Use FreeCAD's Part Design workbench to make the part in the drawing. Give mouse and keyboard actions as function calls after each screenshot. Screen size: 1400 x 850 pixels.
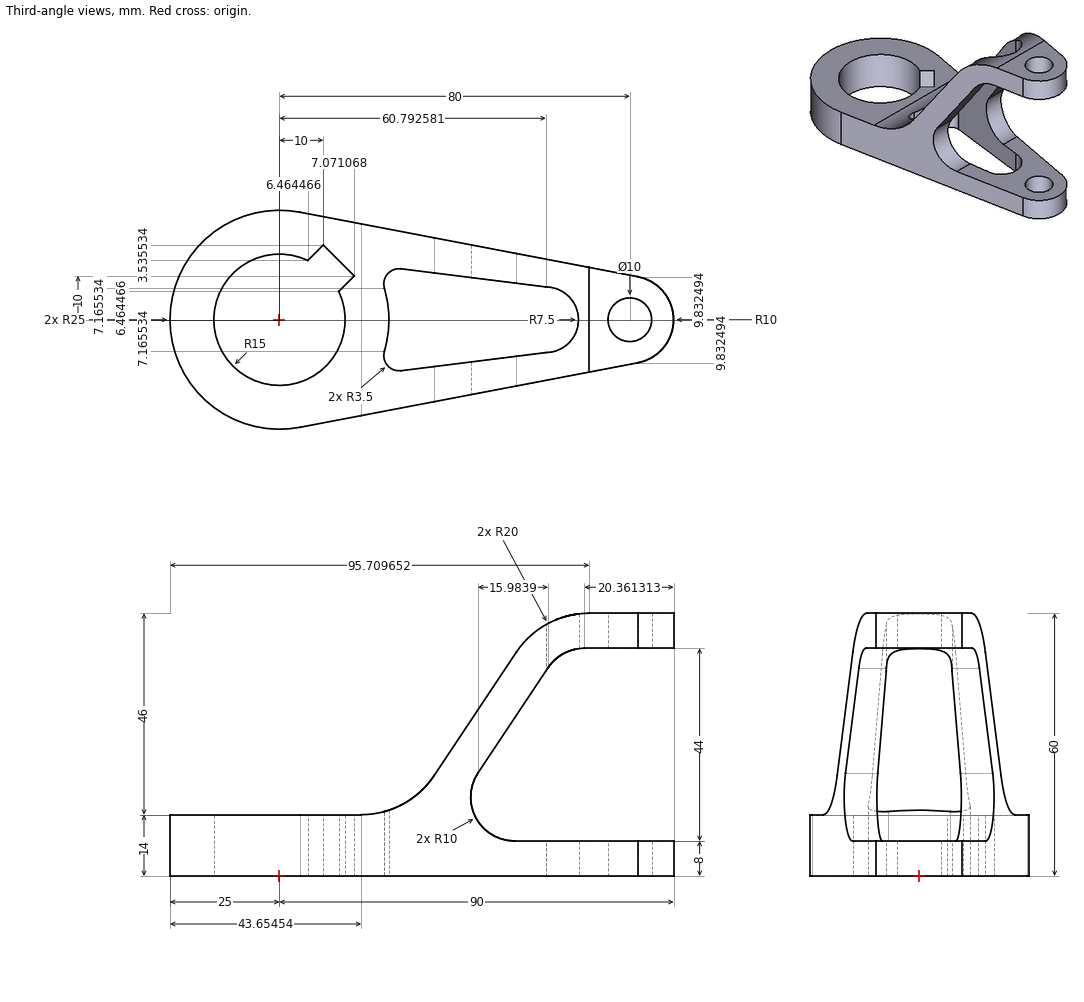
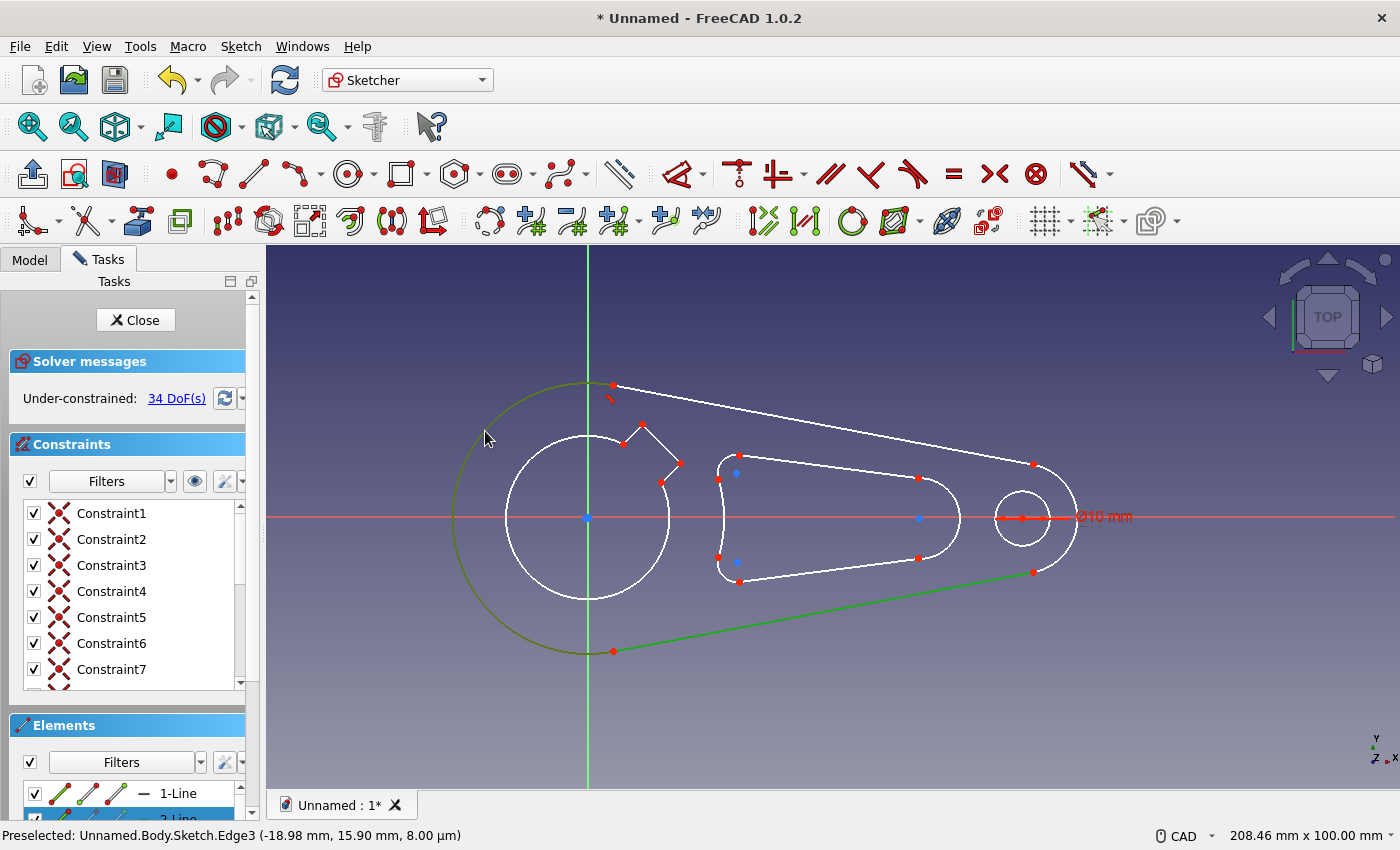
click(913, 174)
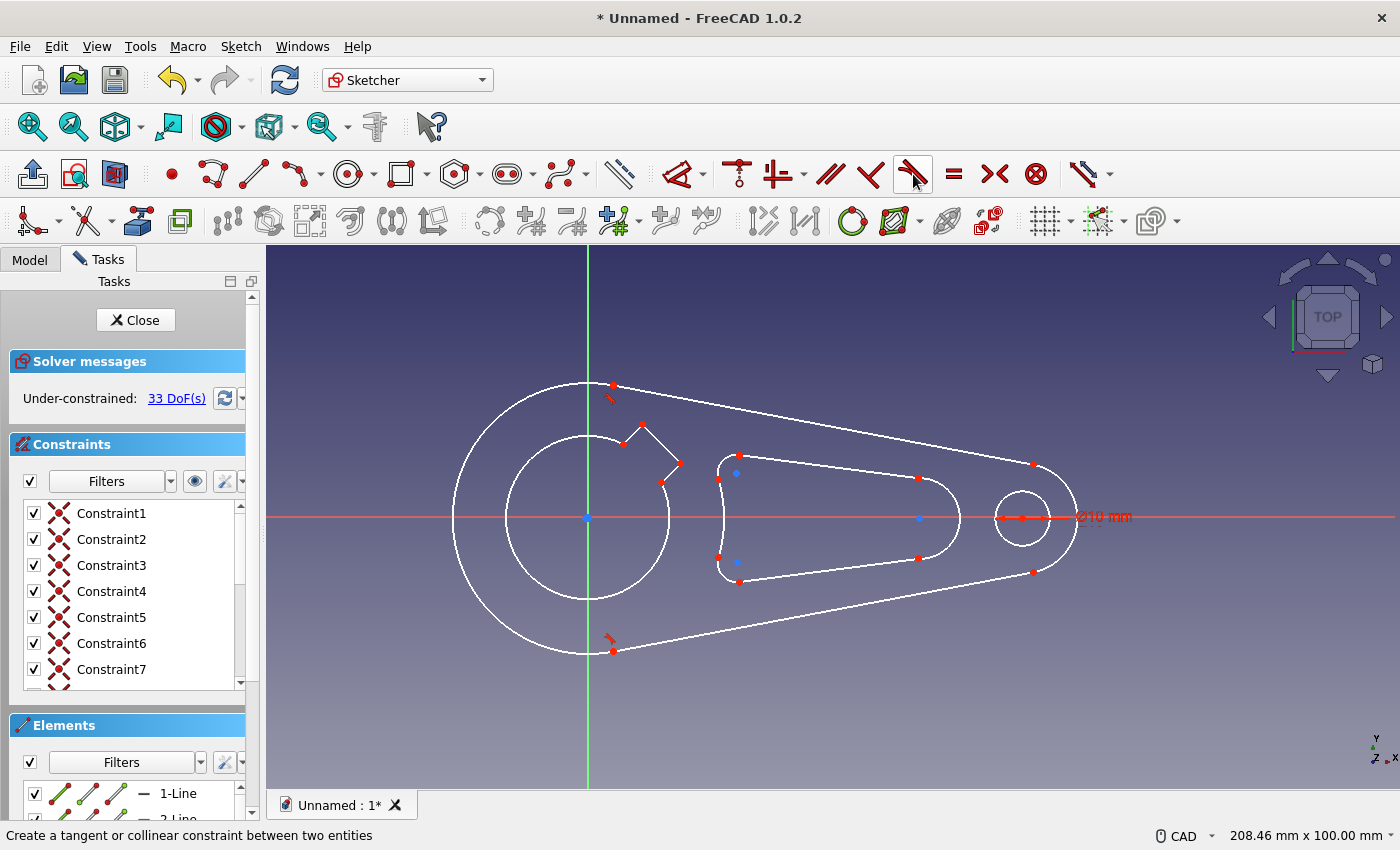
click(793, 462)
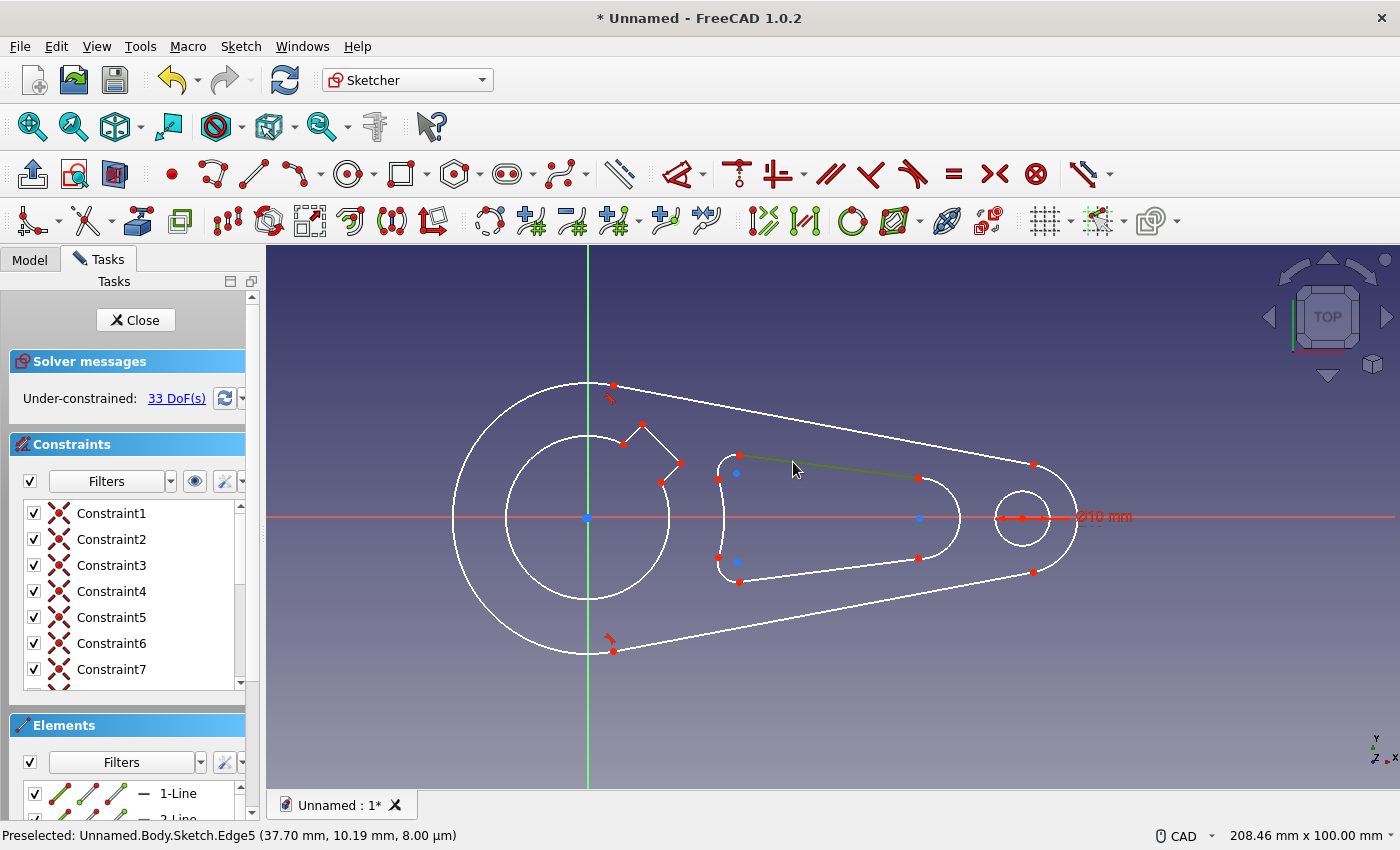
scroll(728, 457, up, 2)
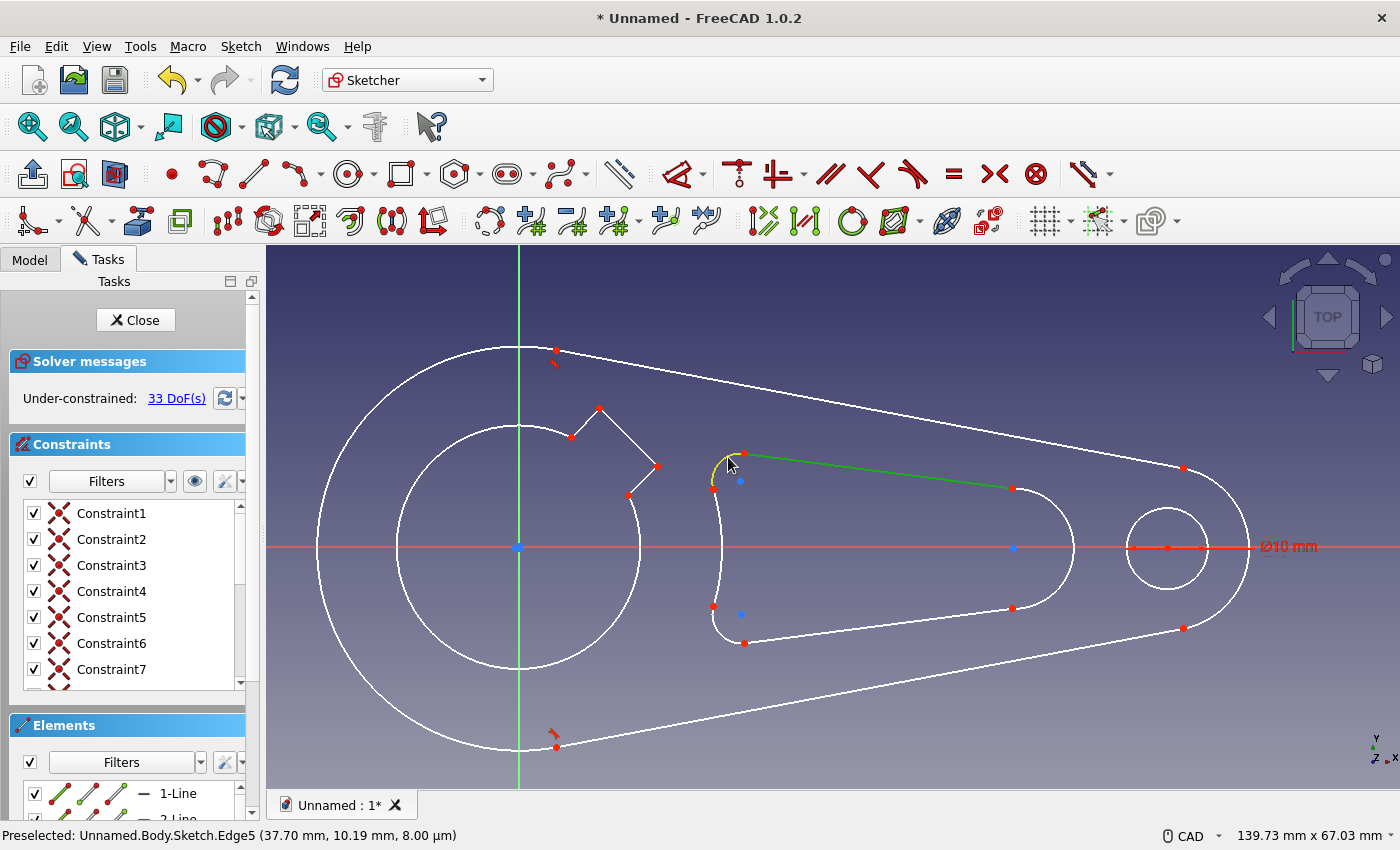
click(728, 456)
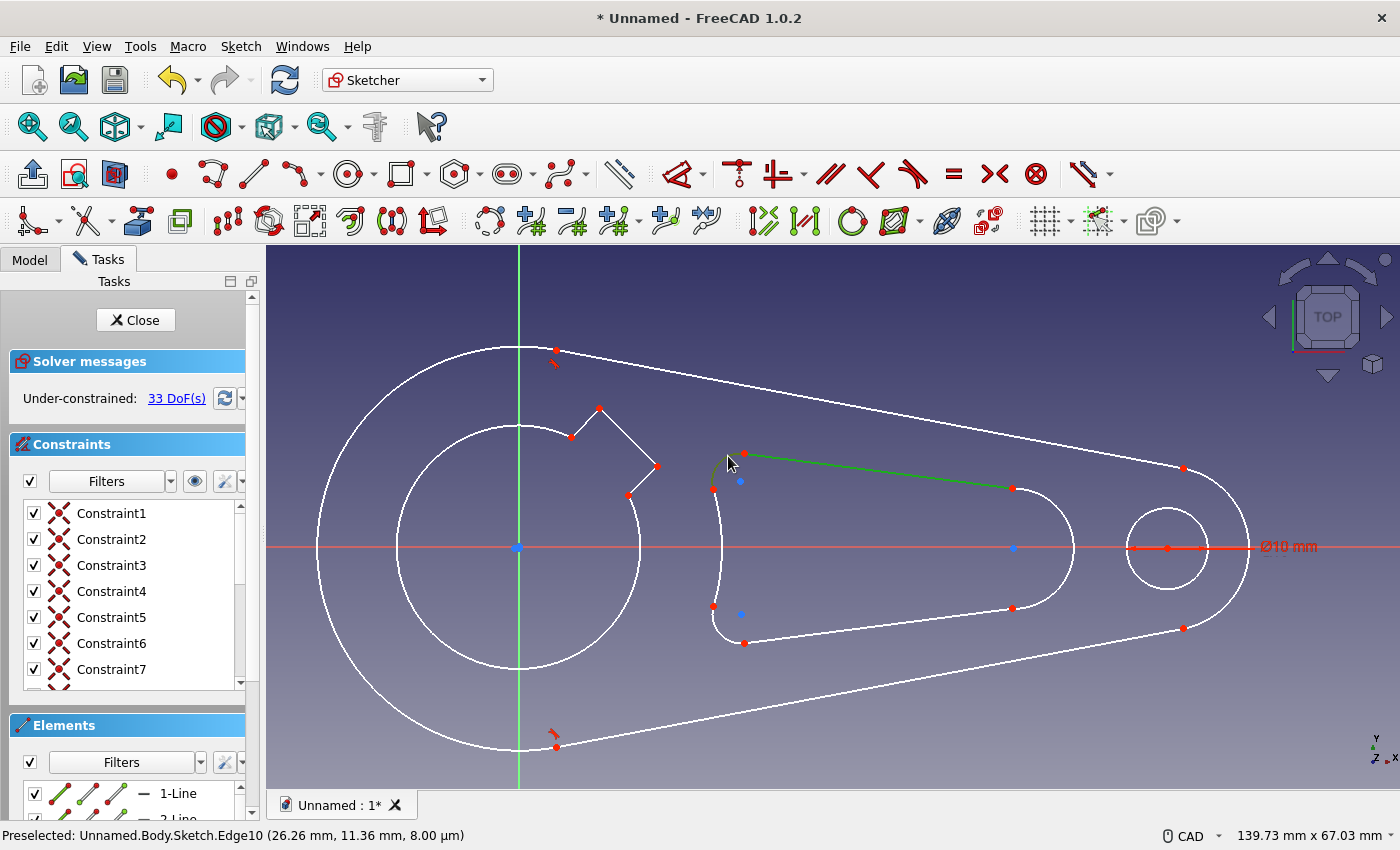
click(913, 174)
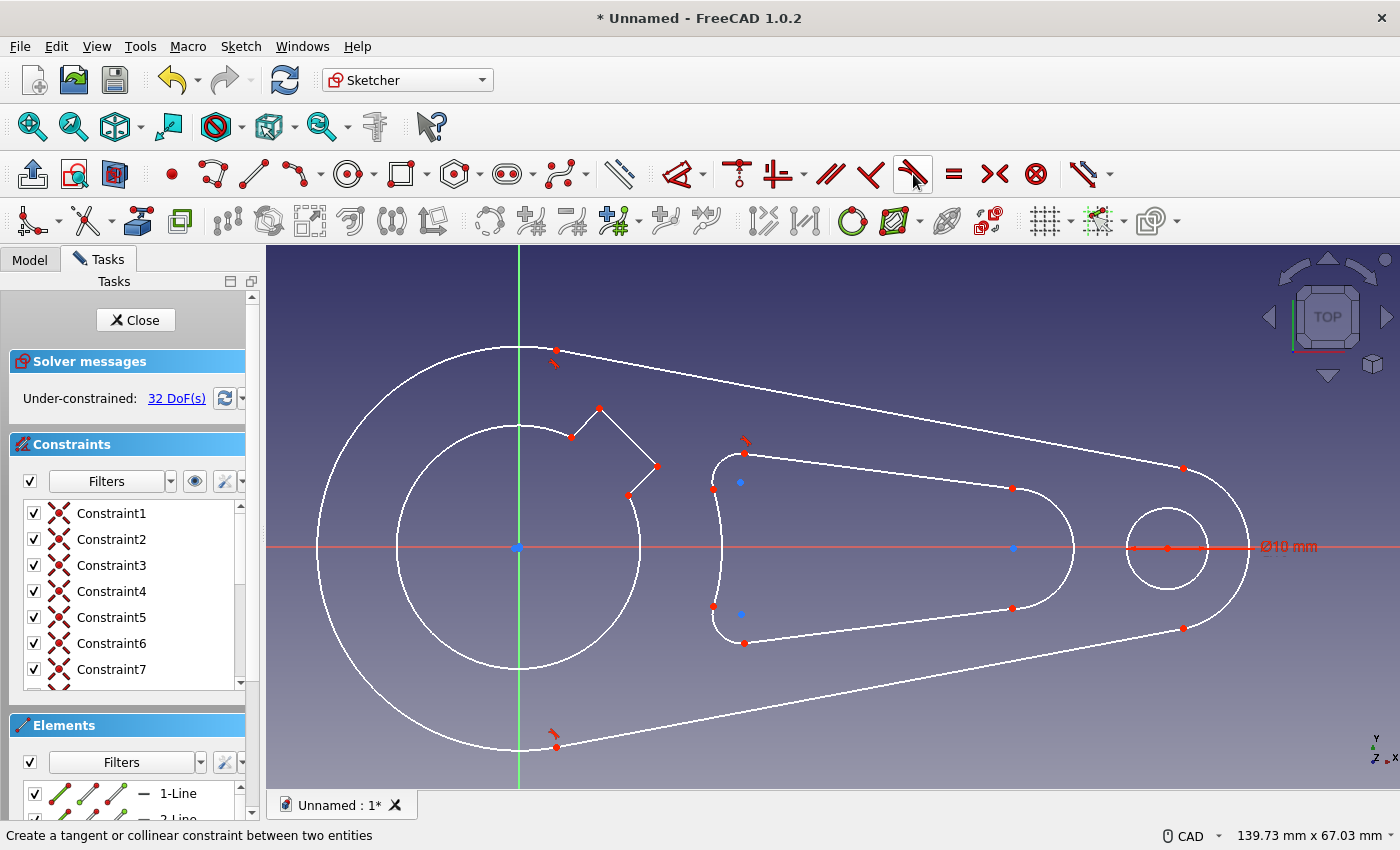
click(932, 619)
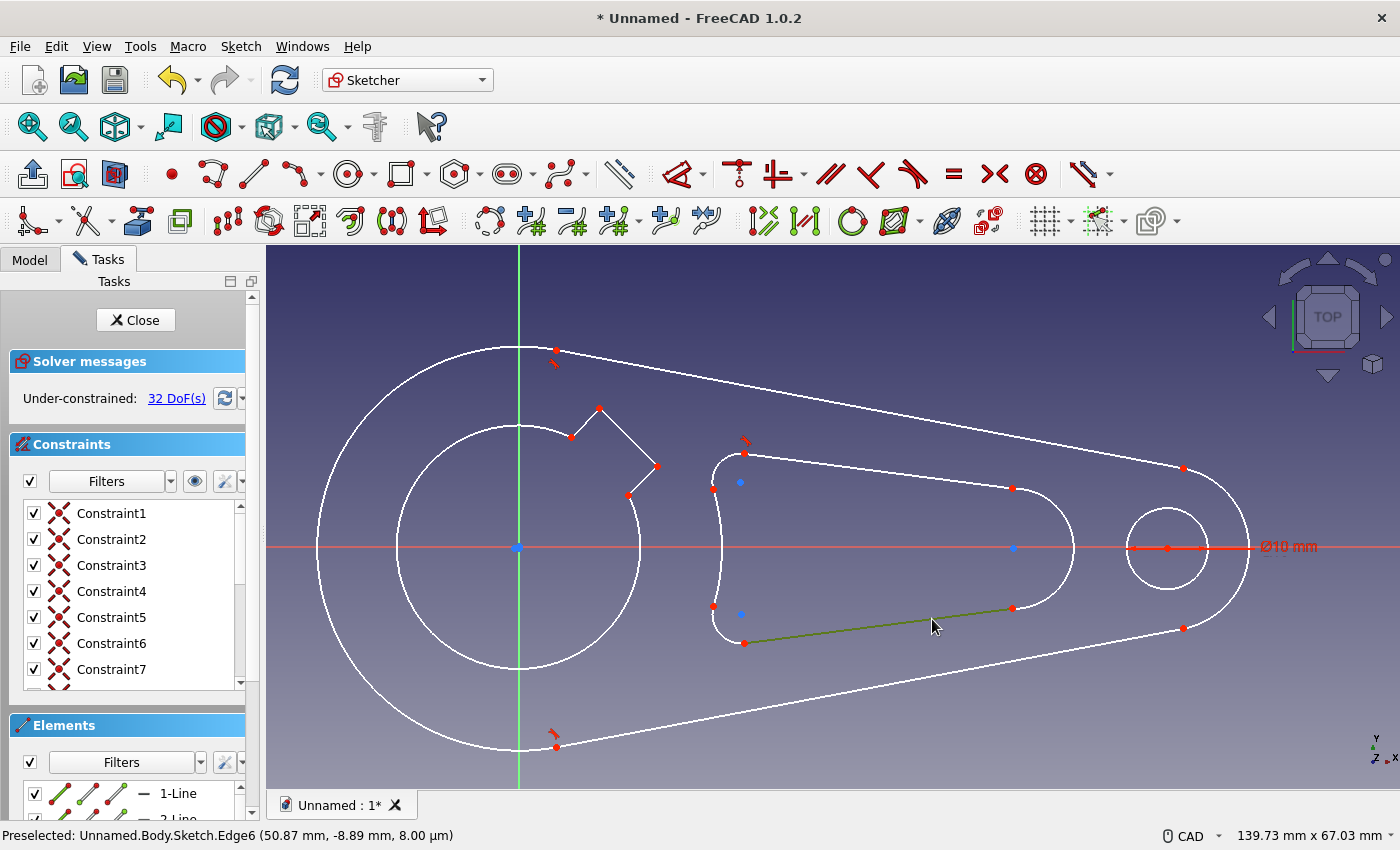
click(714, 624)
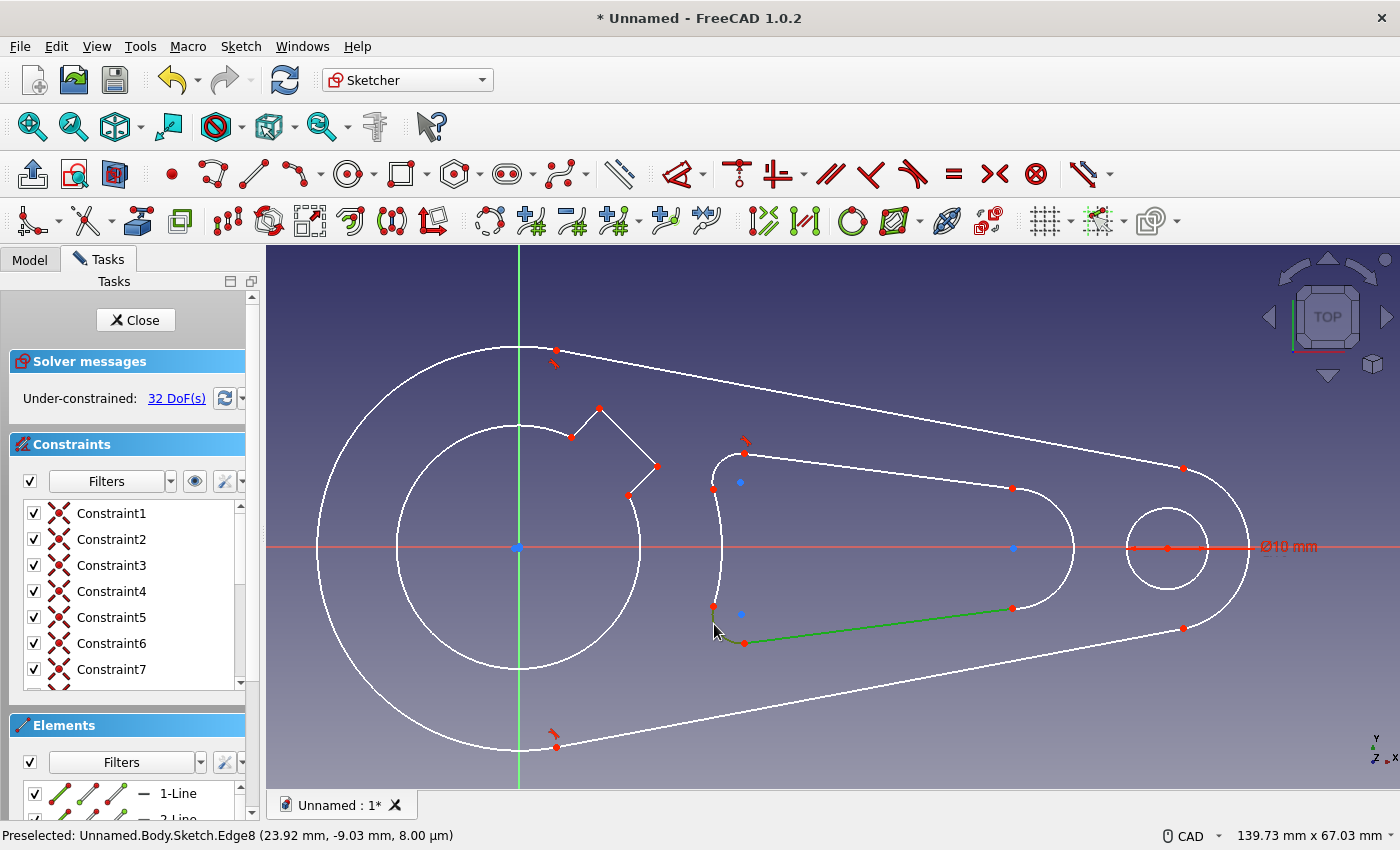
key(t)